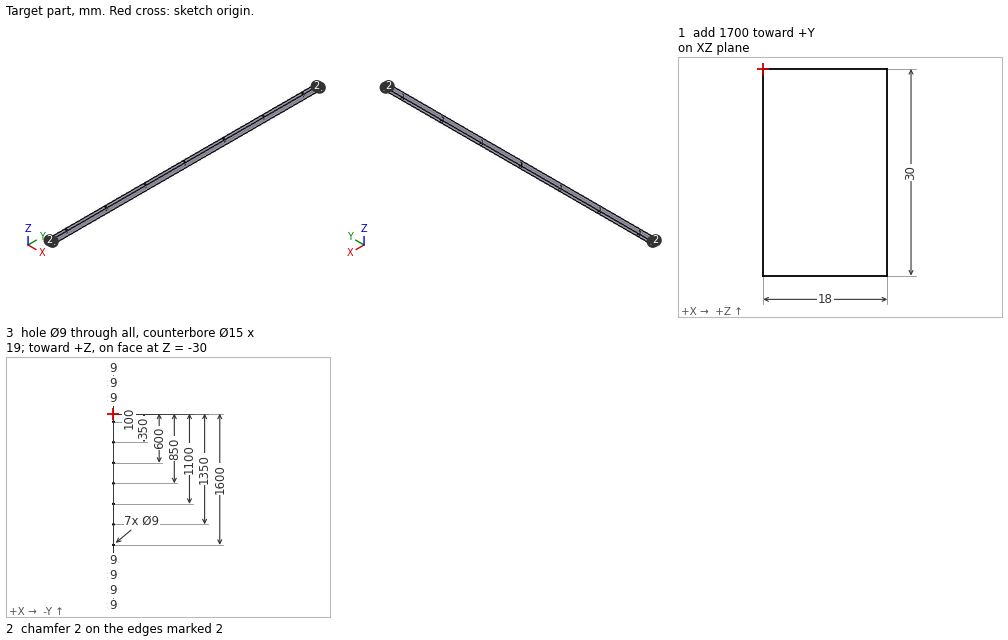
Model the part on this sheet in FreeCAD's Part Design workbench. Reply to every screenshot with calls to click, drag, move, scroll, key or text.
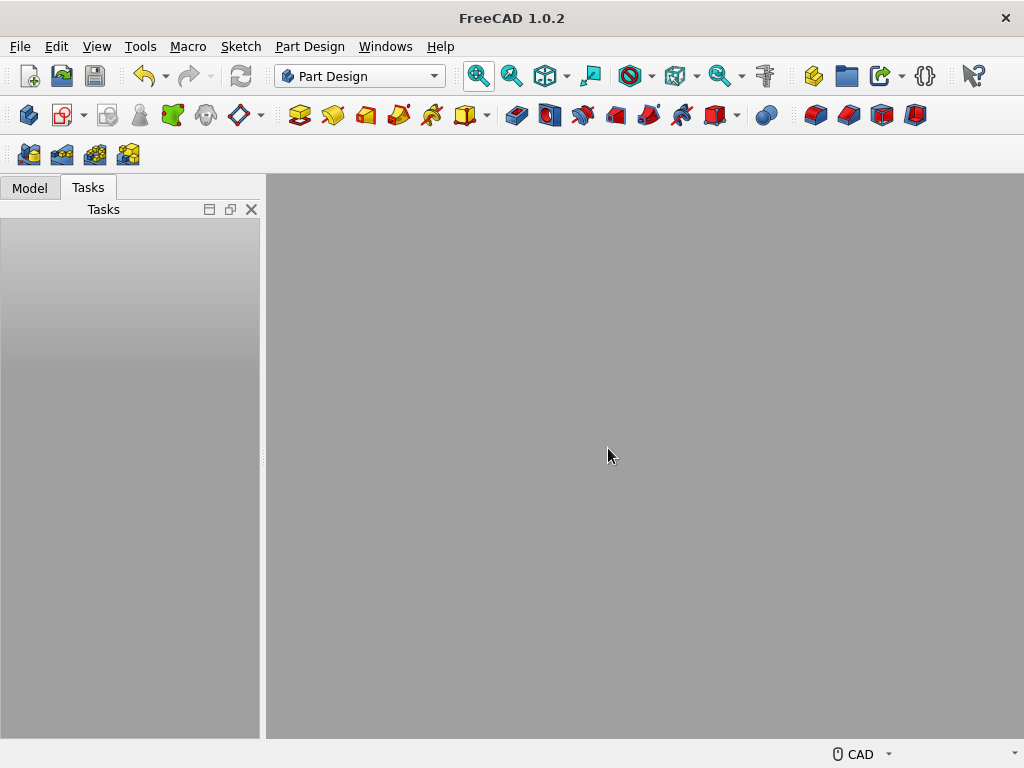
key(ctrl+n)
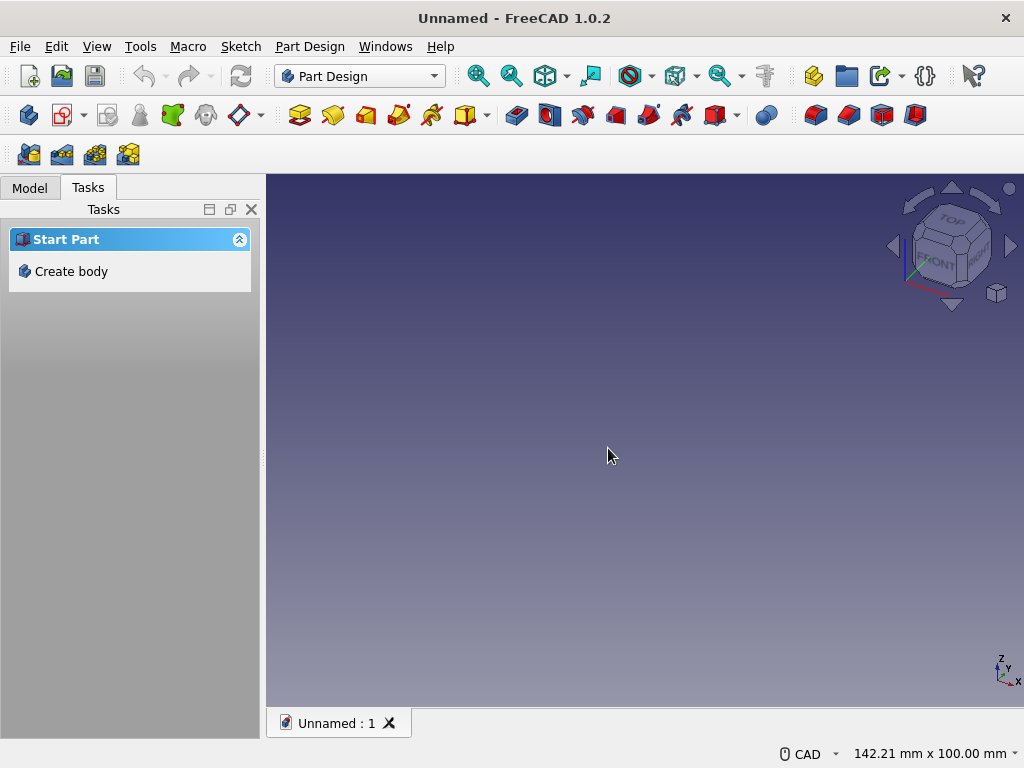
click(62, 116)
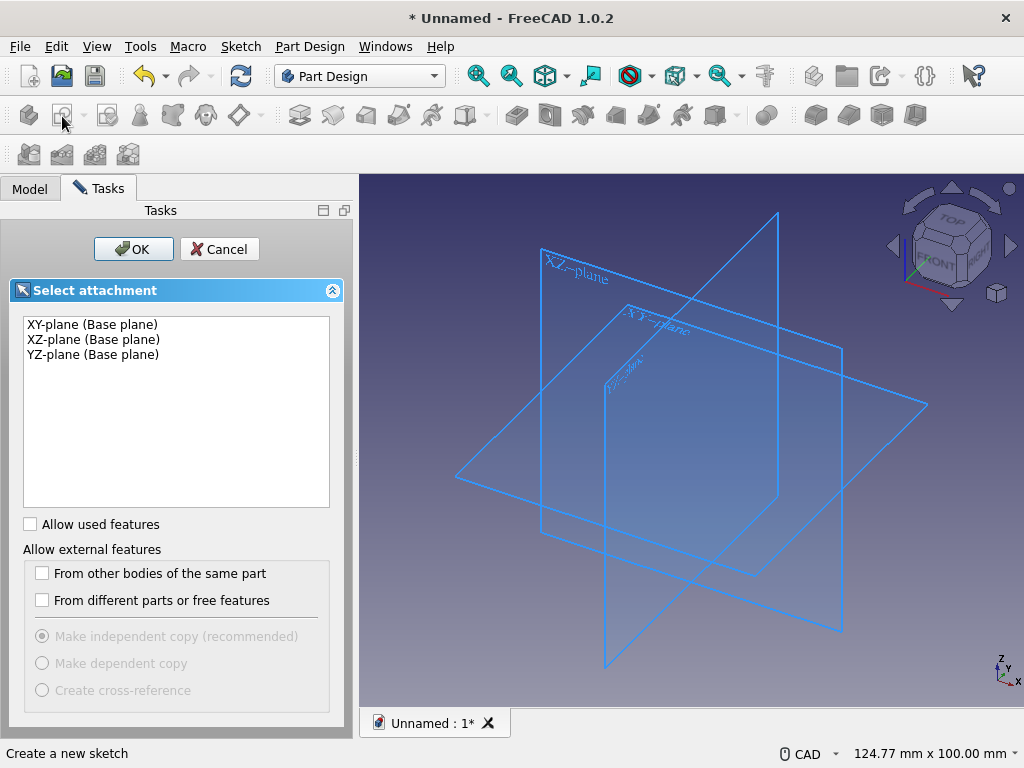
click(84, 340)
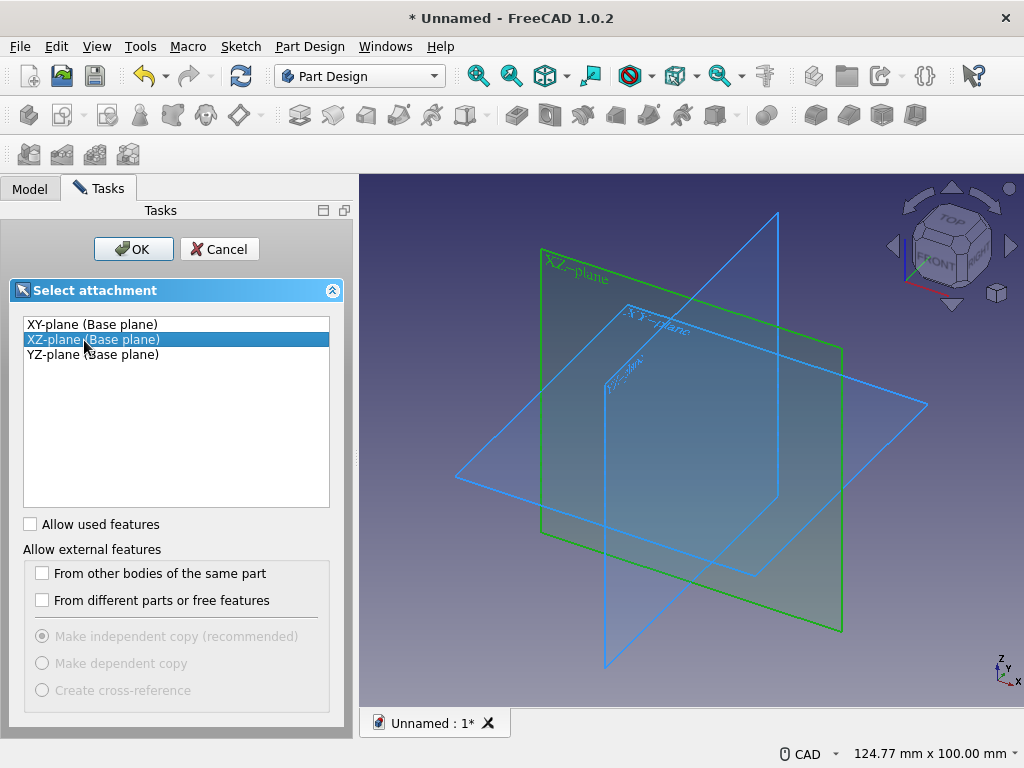
click(134, 249)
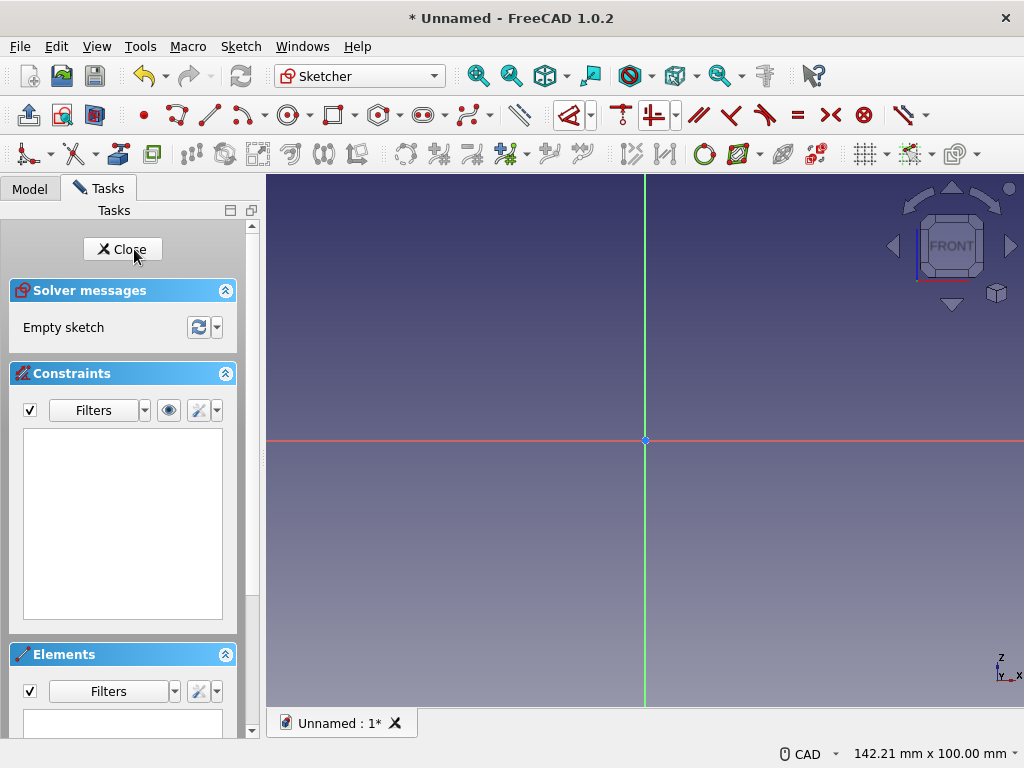
scroll(788, 586, up, 4)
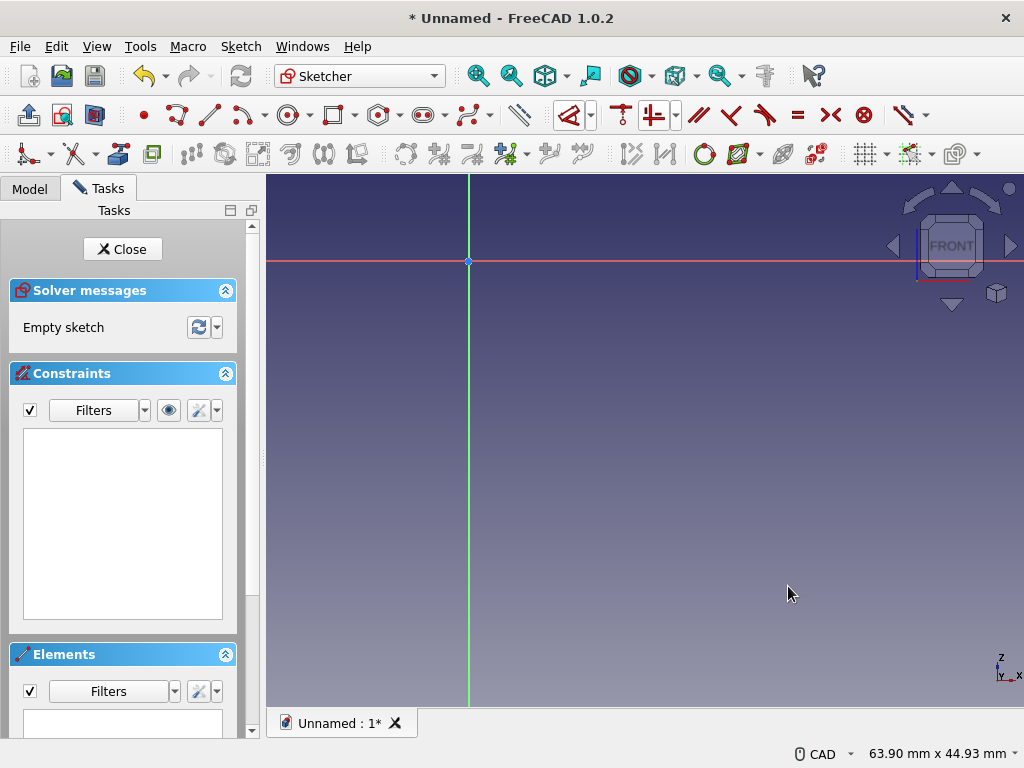
key(g)
key(r)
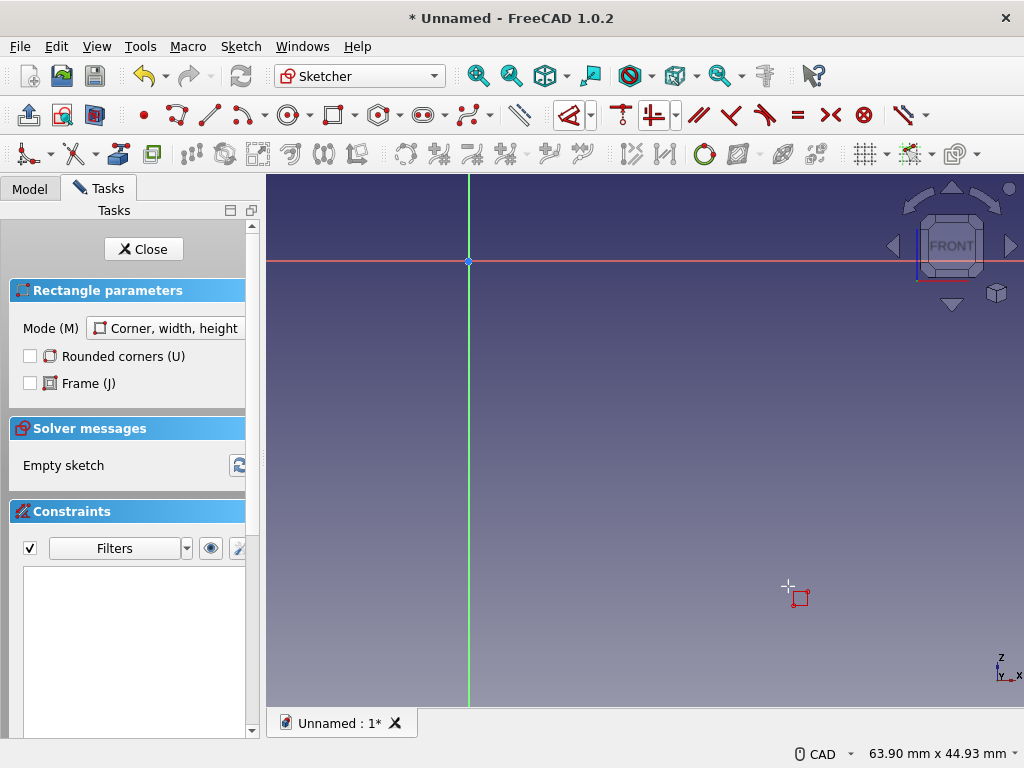
click(469, 261)
move(682, 617)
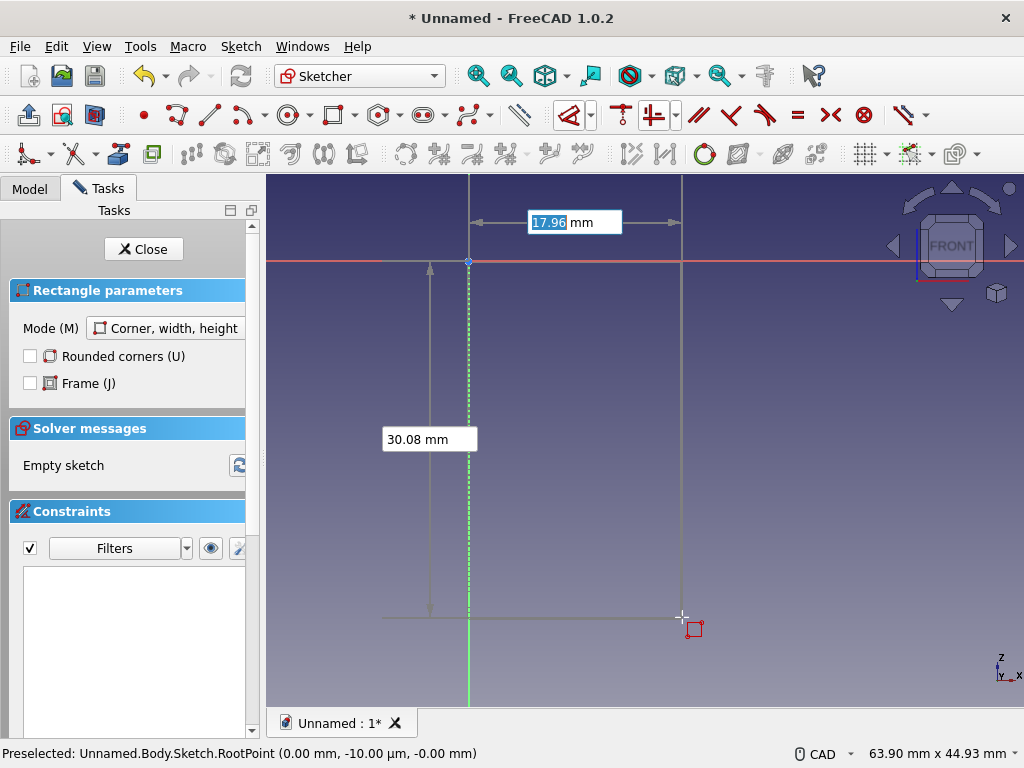
text(18)
key(Tab)
text(30)
key(Return)
key(Escape)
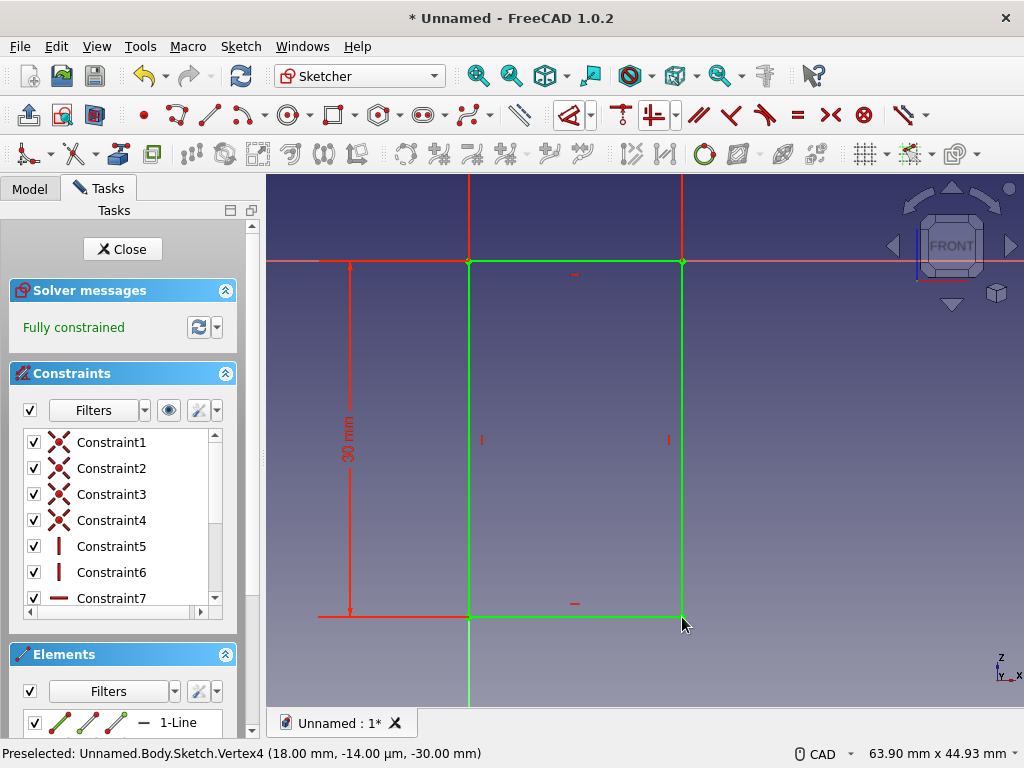
click(123, 249)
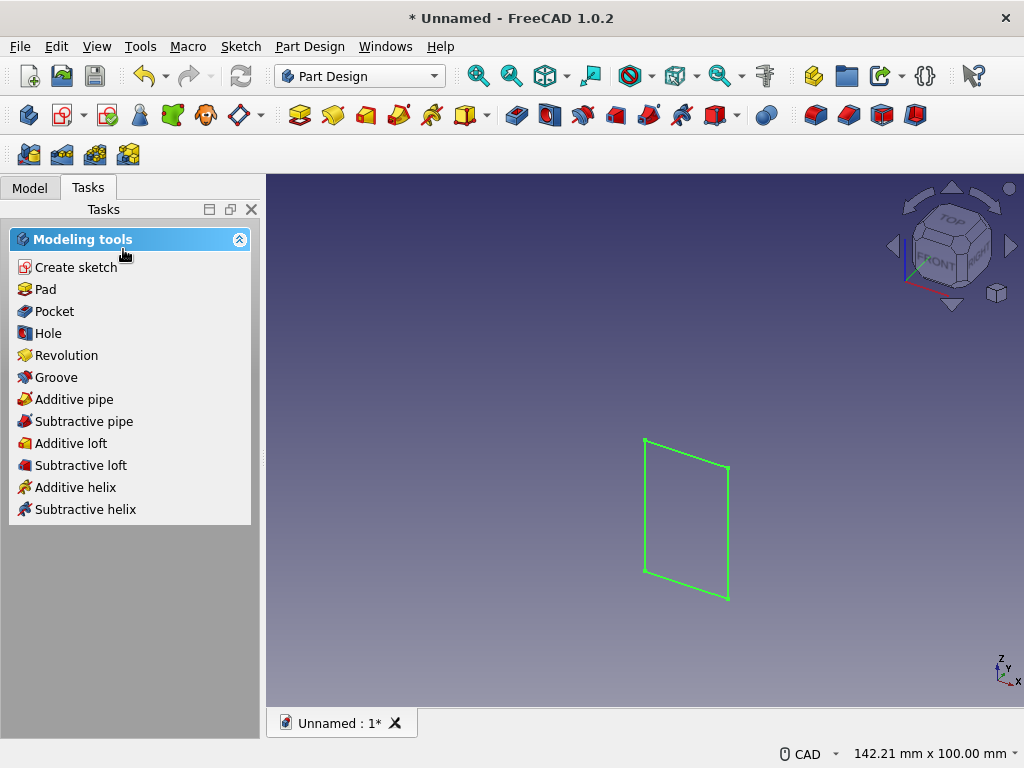
click(300, 116)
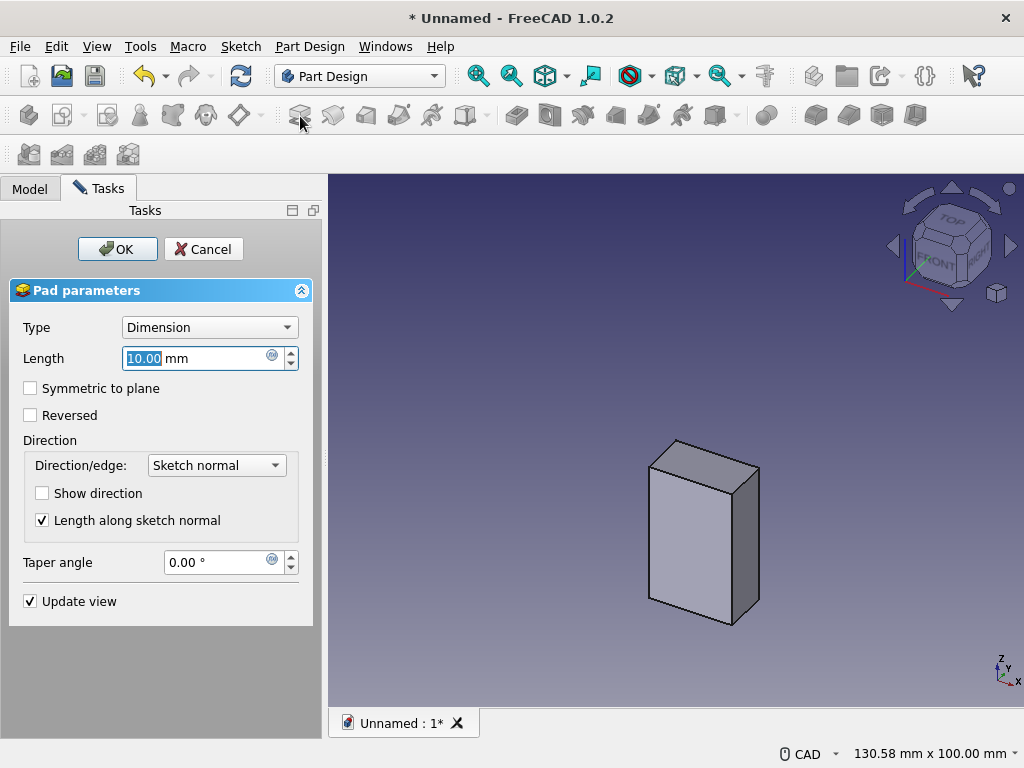
text(1700)
key(Tab)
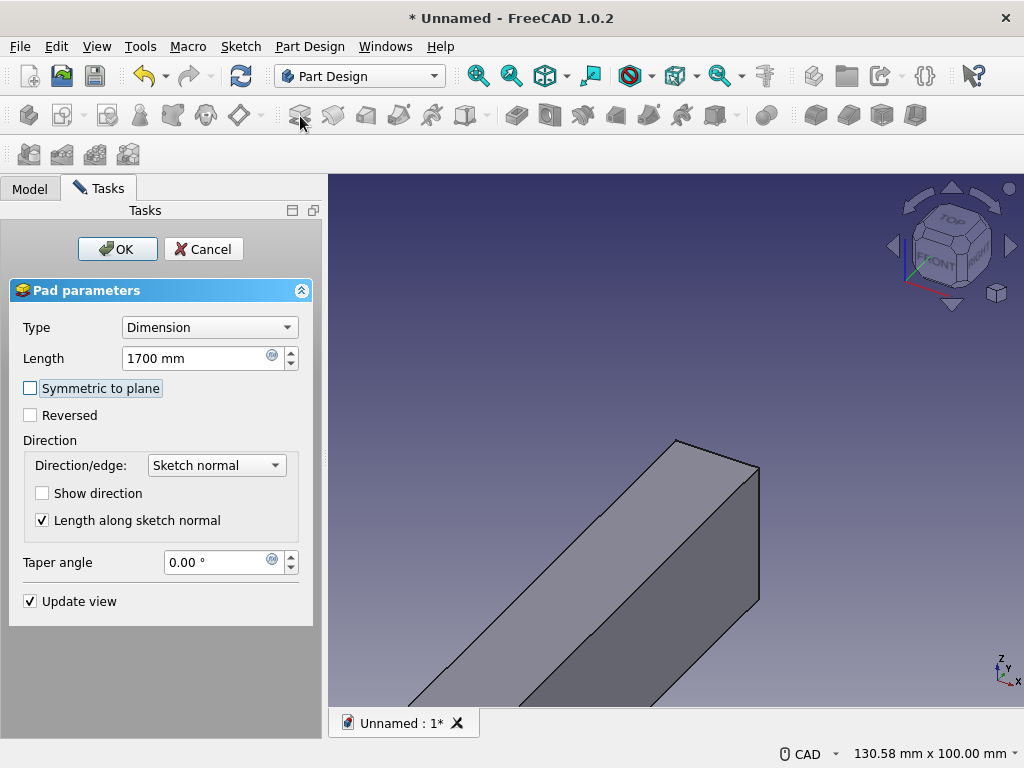
click(31, 415)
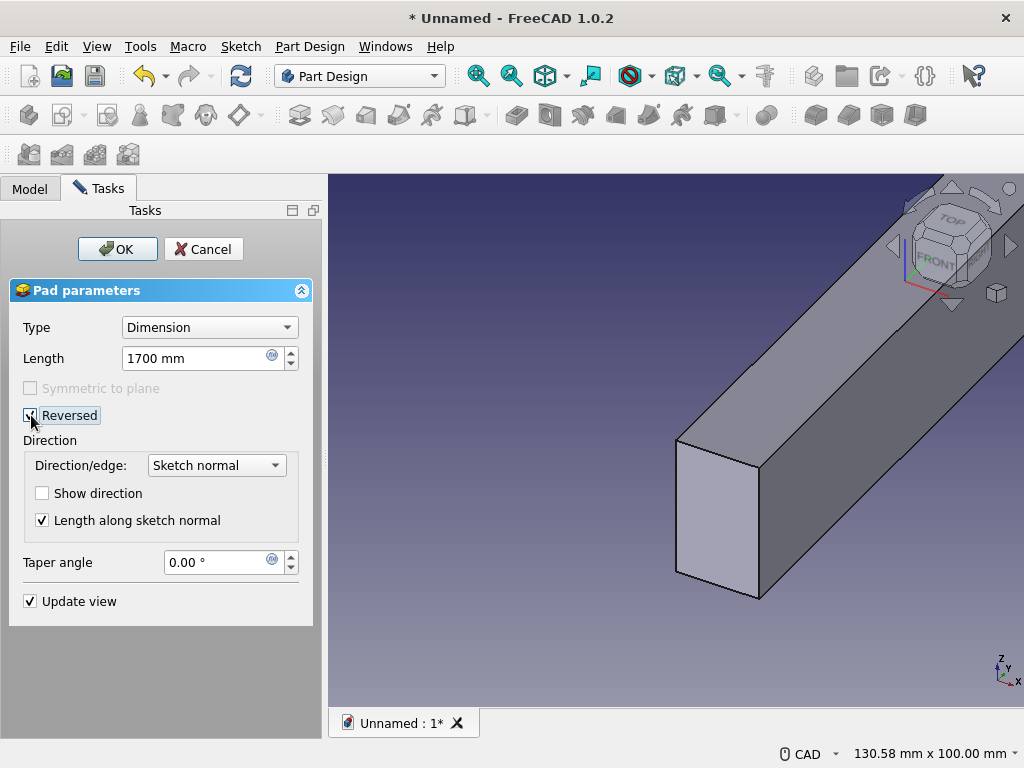
click(118, 249)